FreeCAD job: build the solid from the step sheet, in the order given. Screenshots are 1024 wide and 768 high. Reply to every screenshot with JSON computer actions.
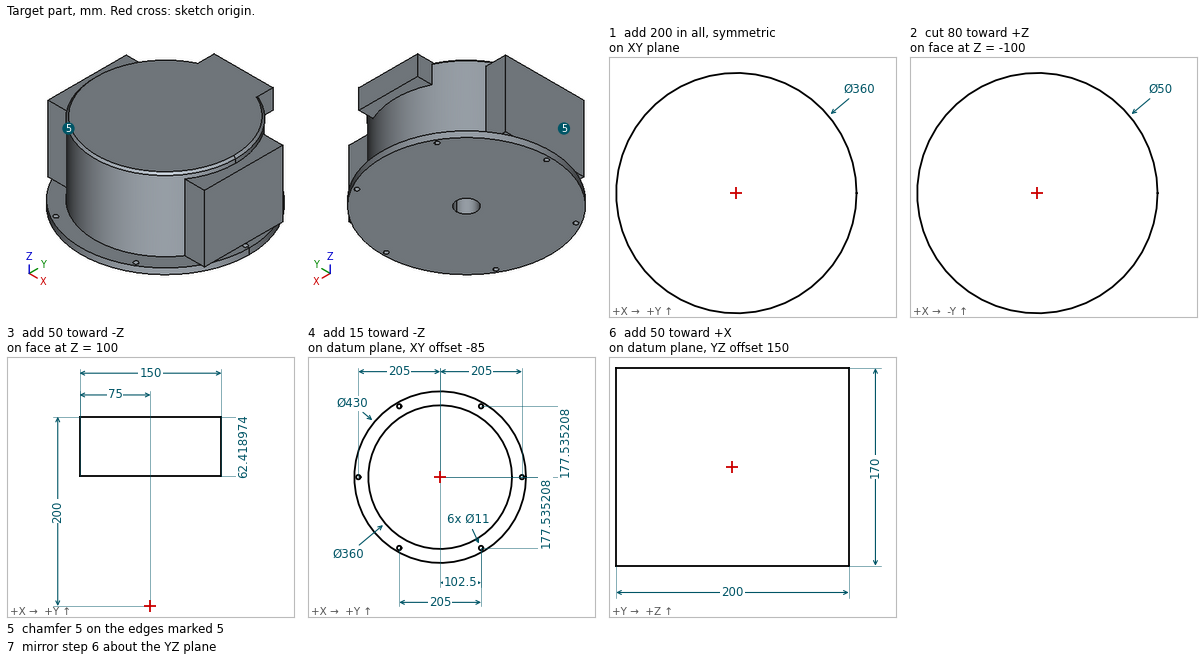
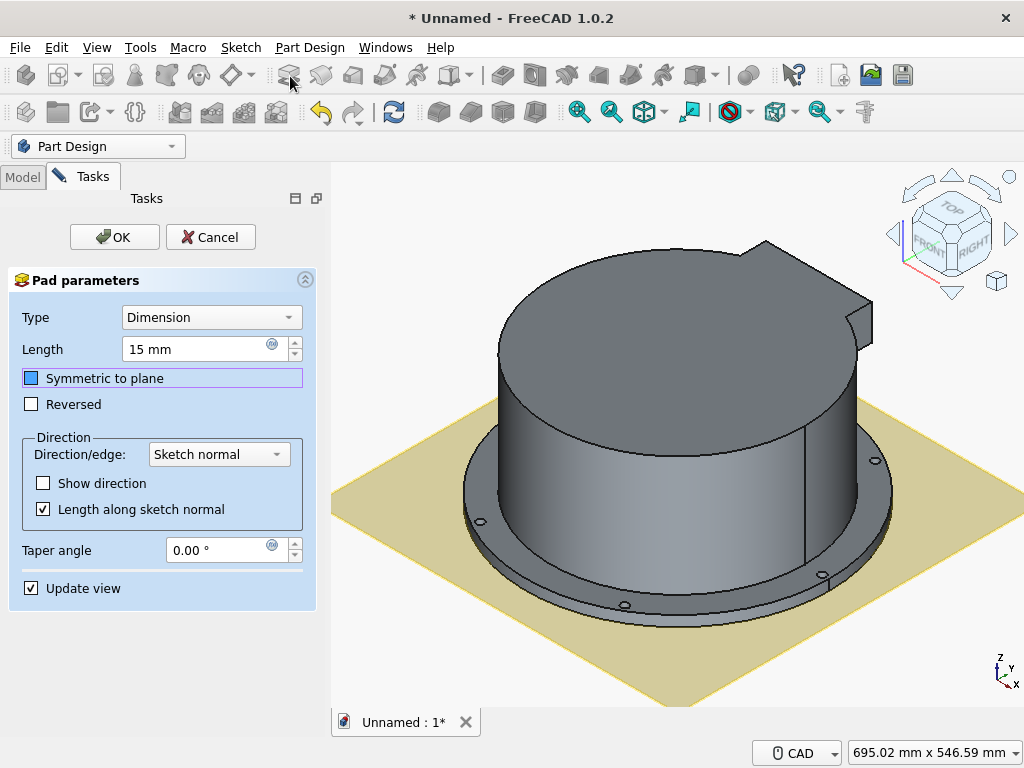
{"action": "left_click", "coordinate": [30, 404]}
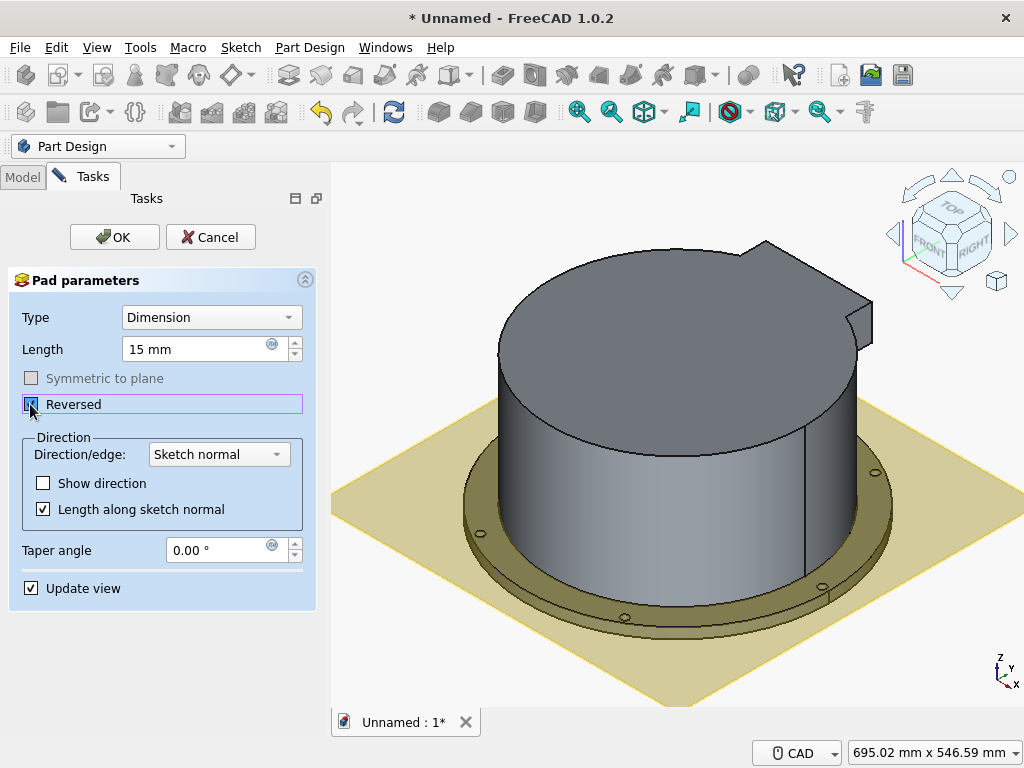
{"action": "left_click", "coordinate": [115, 237]}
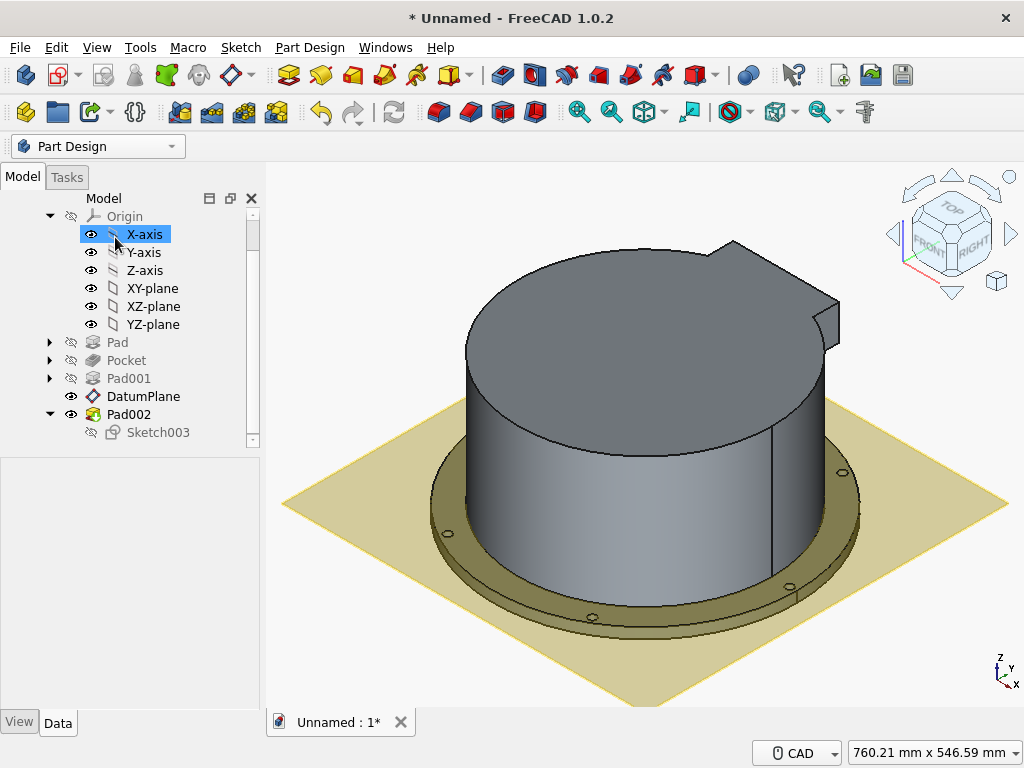
{"action": "left_click", "coordinate": [116, 396]}
{"action": "key", "text": "space"}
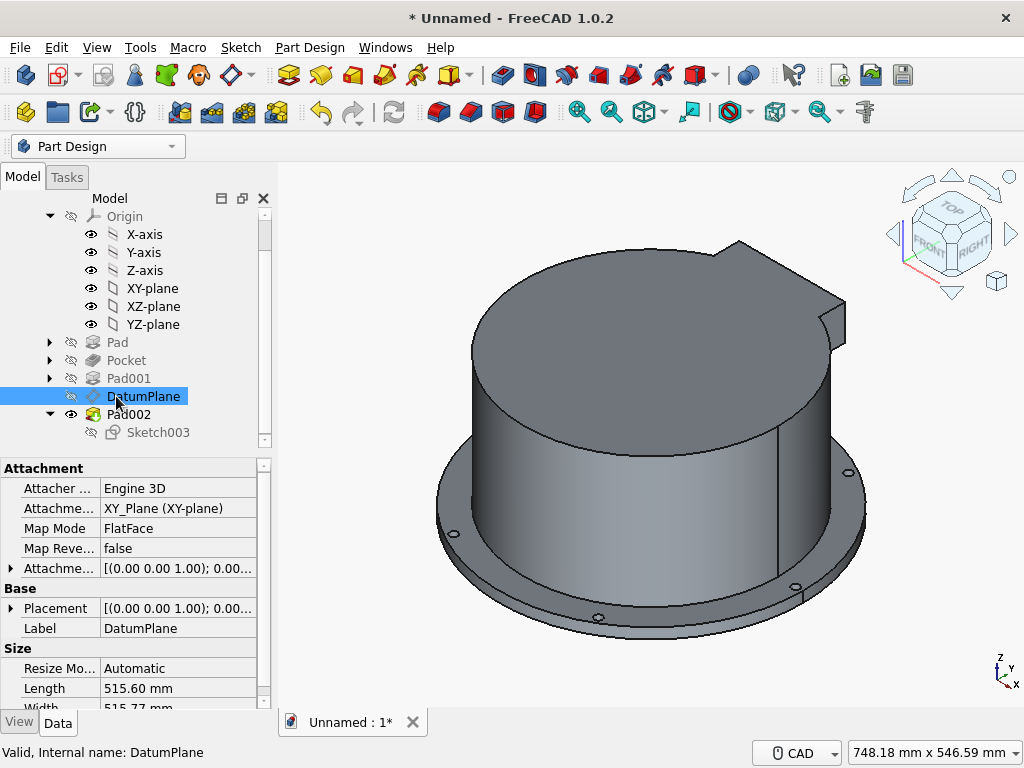
{"action": "left_click", "coordinate": [476, 374]}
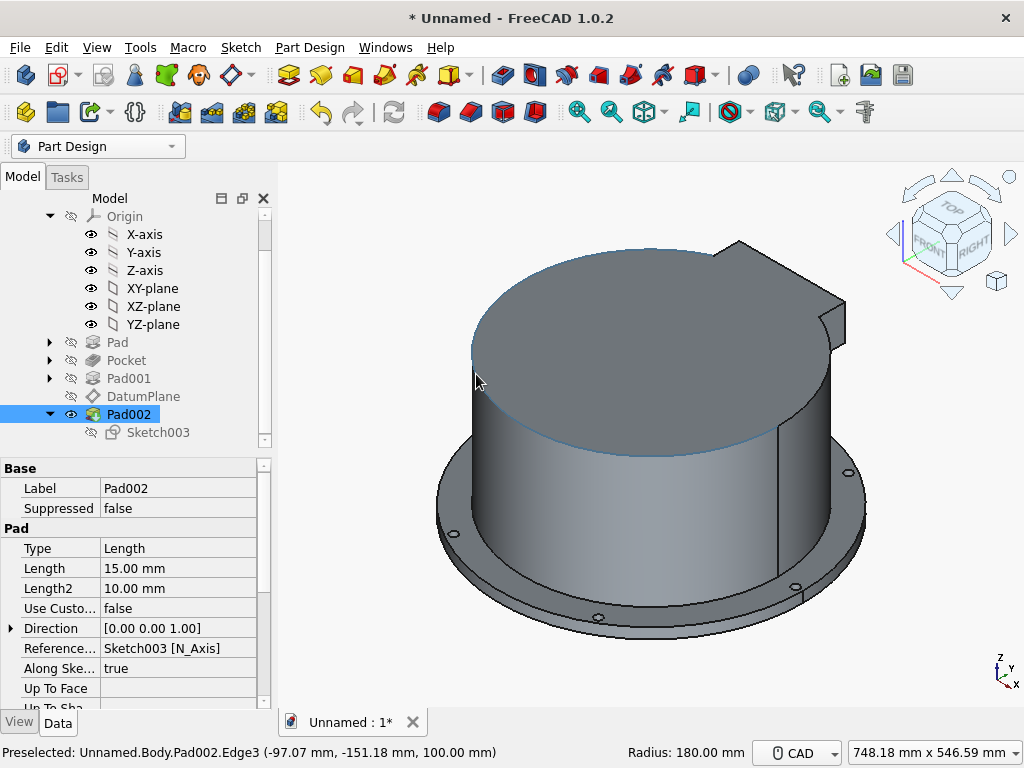
{"action": "left_click", "coordinate": [472, 112]}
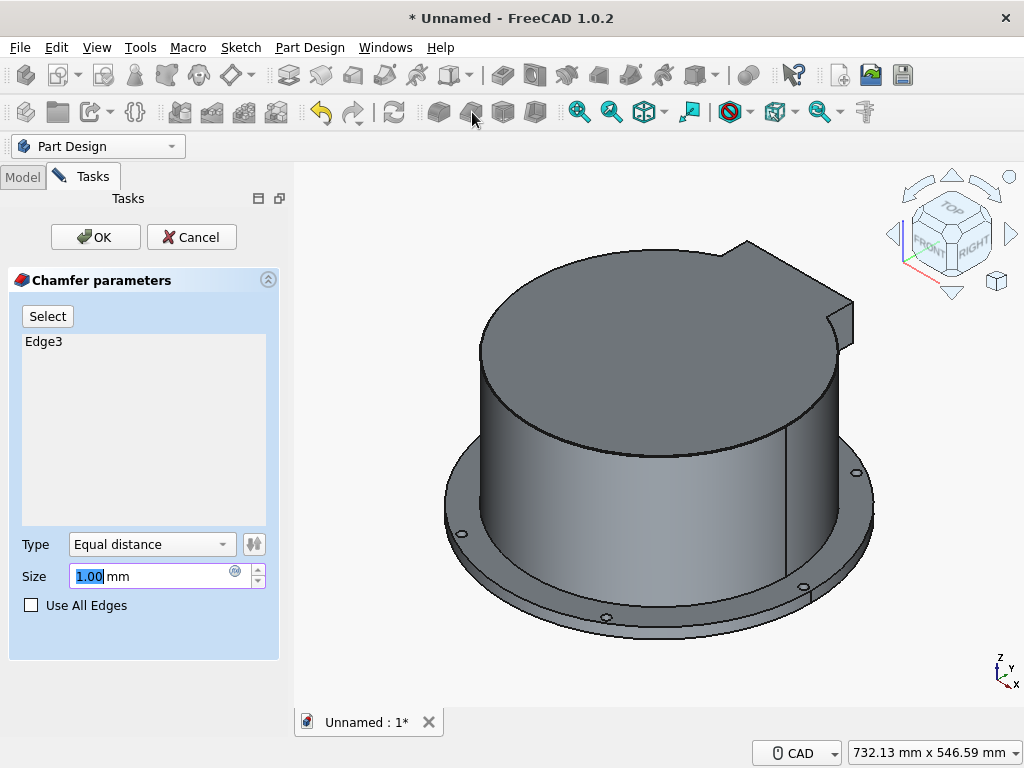
{"action": "type", "text": "5"}
{"action": "key", "text": "Tab"}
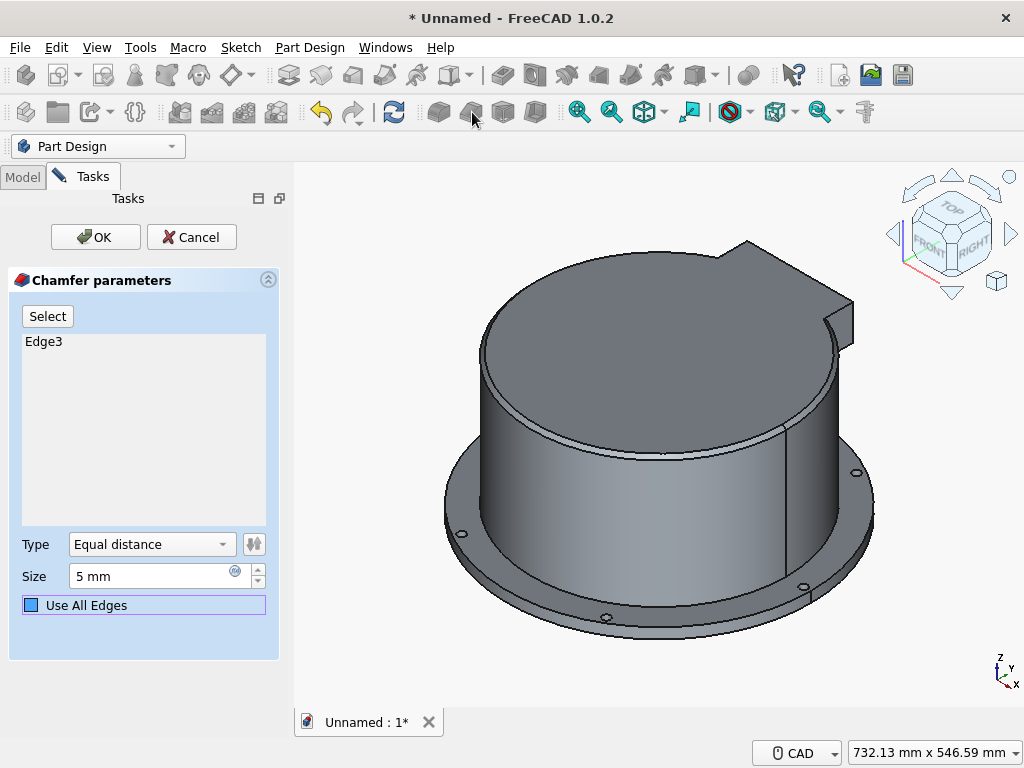
{"action": "left_click", "coordinate": [96, 237]}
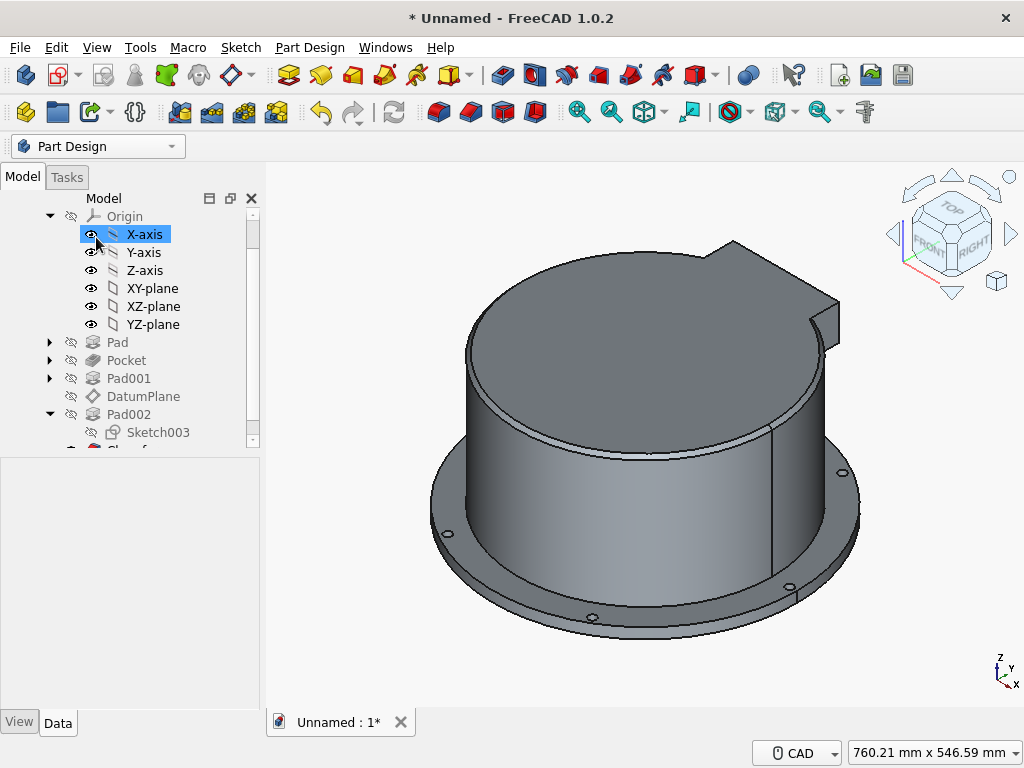
{"action": "left_click", "coordinate": [136, 324]}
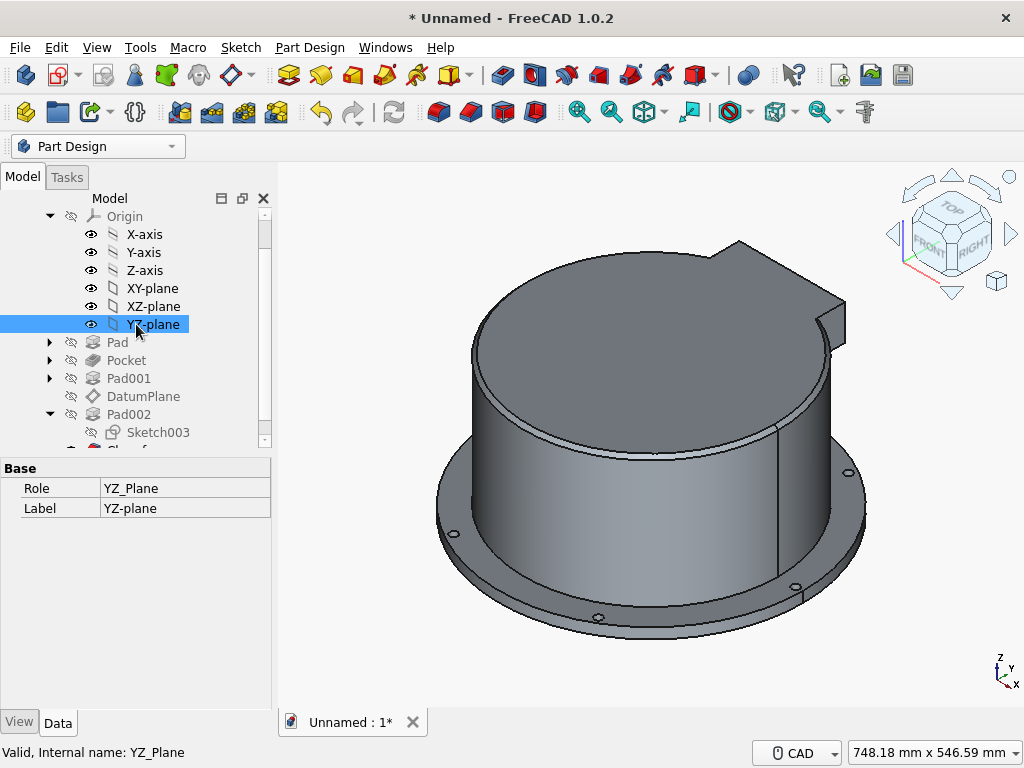
{"action": "left_click", "coordinate": [232, 76]}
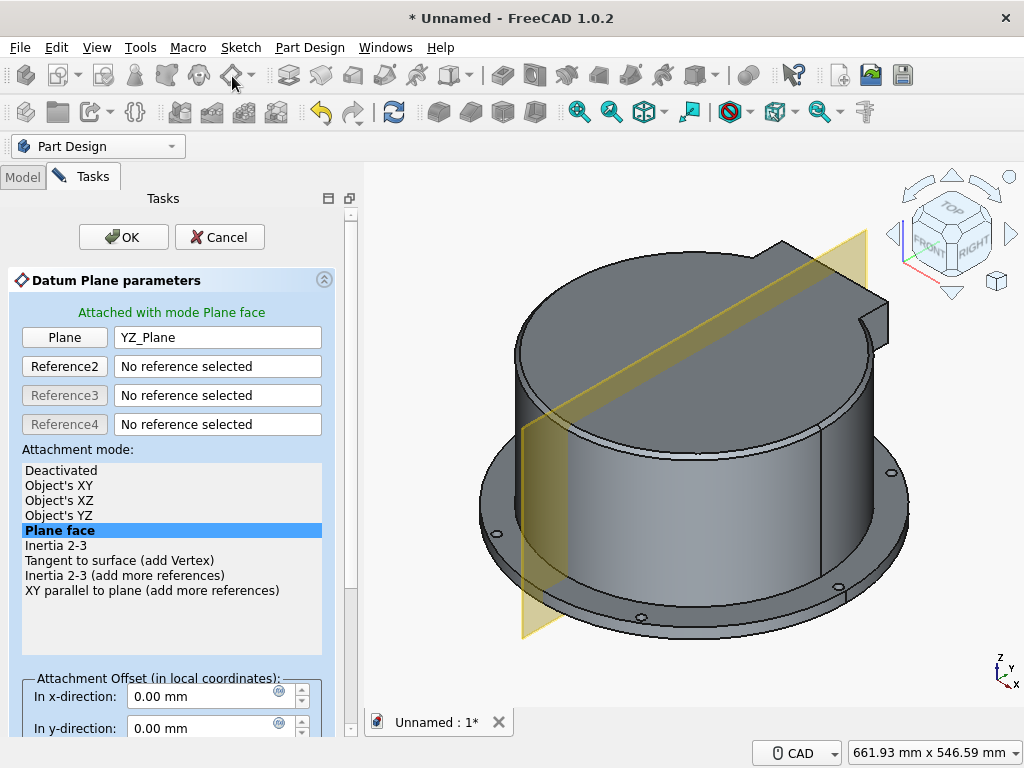
{"action": "scroll", "coordinate": [351, 472], "scroll_direction": "down", "scroll_amount": 2}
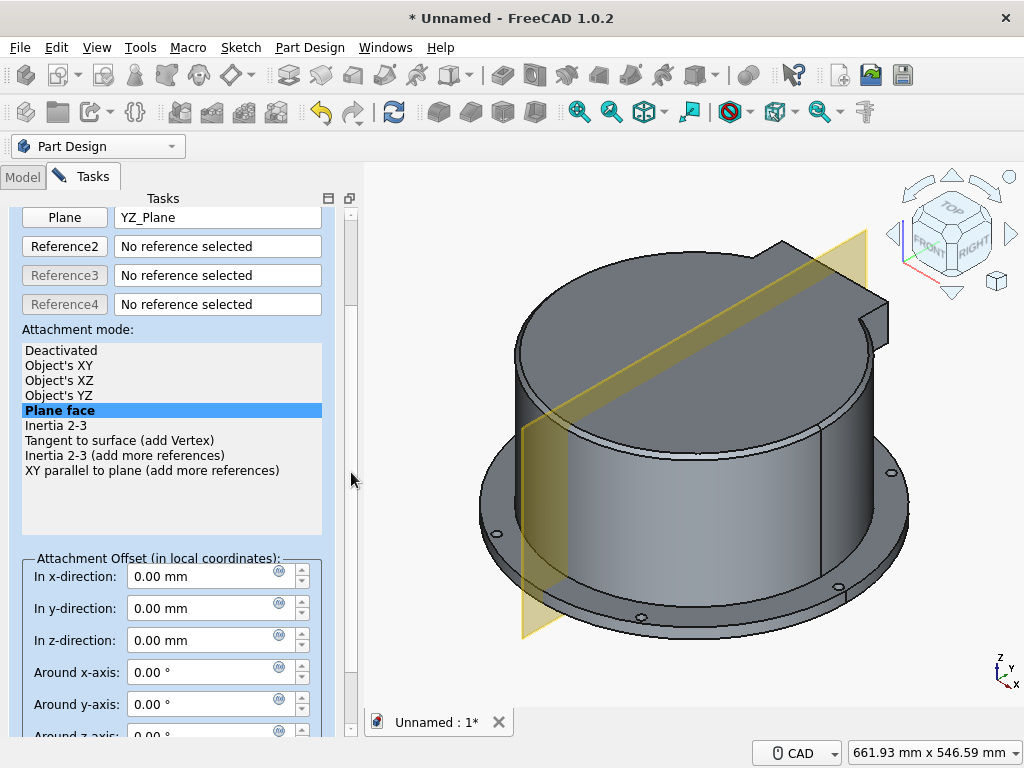
{"action": "triple_click", "coordinate": [210, 640]}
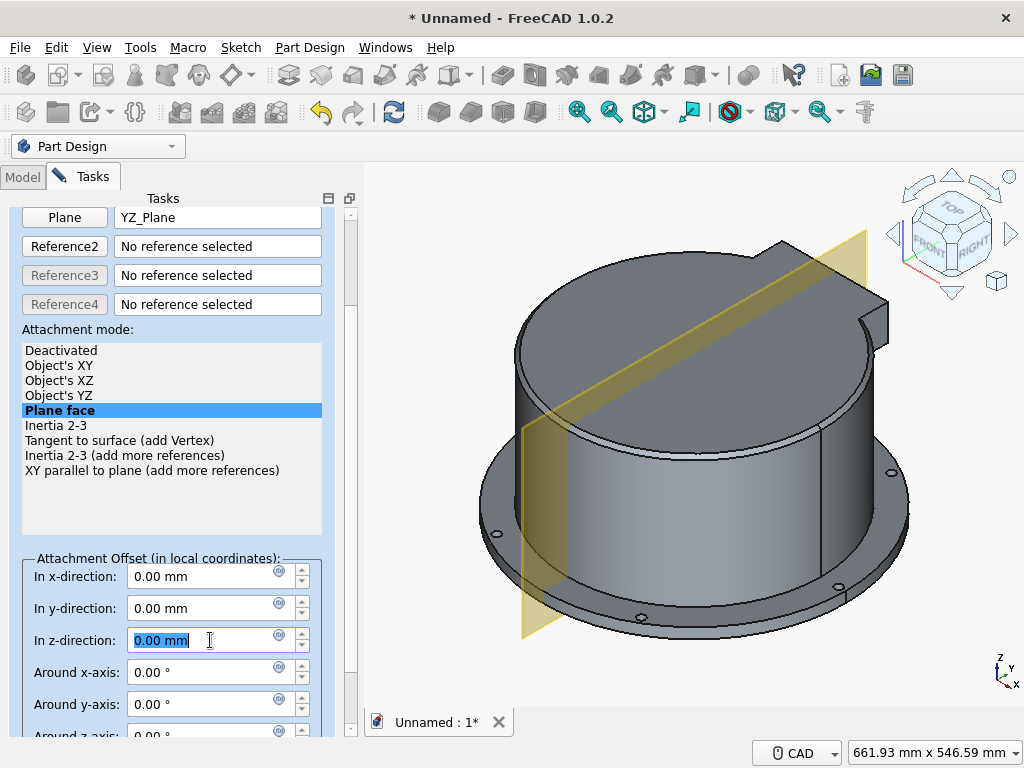
{"action": "type", "text": "150"}
{"action": "key", "text": "Tab"}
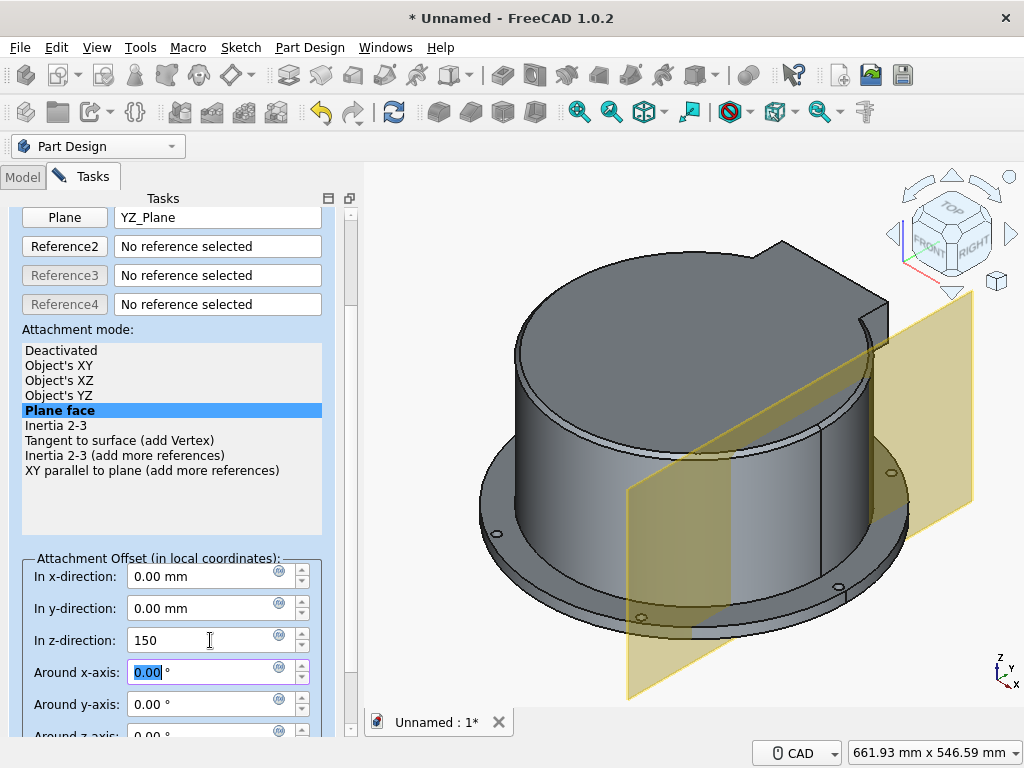
{"action": "scroll", "coordinate": [351, 472], "scroll_direction": "up", "scroll_amount": 3}